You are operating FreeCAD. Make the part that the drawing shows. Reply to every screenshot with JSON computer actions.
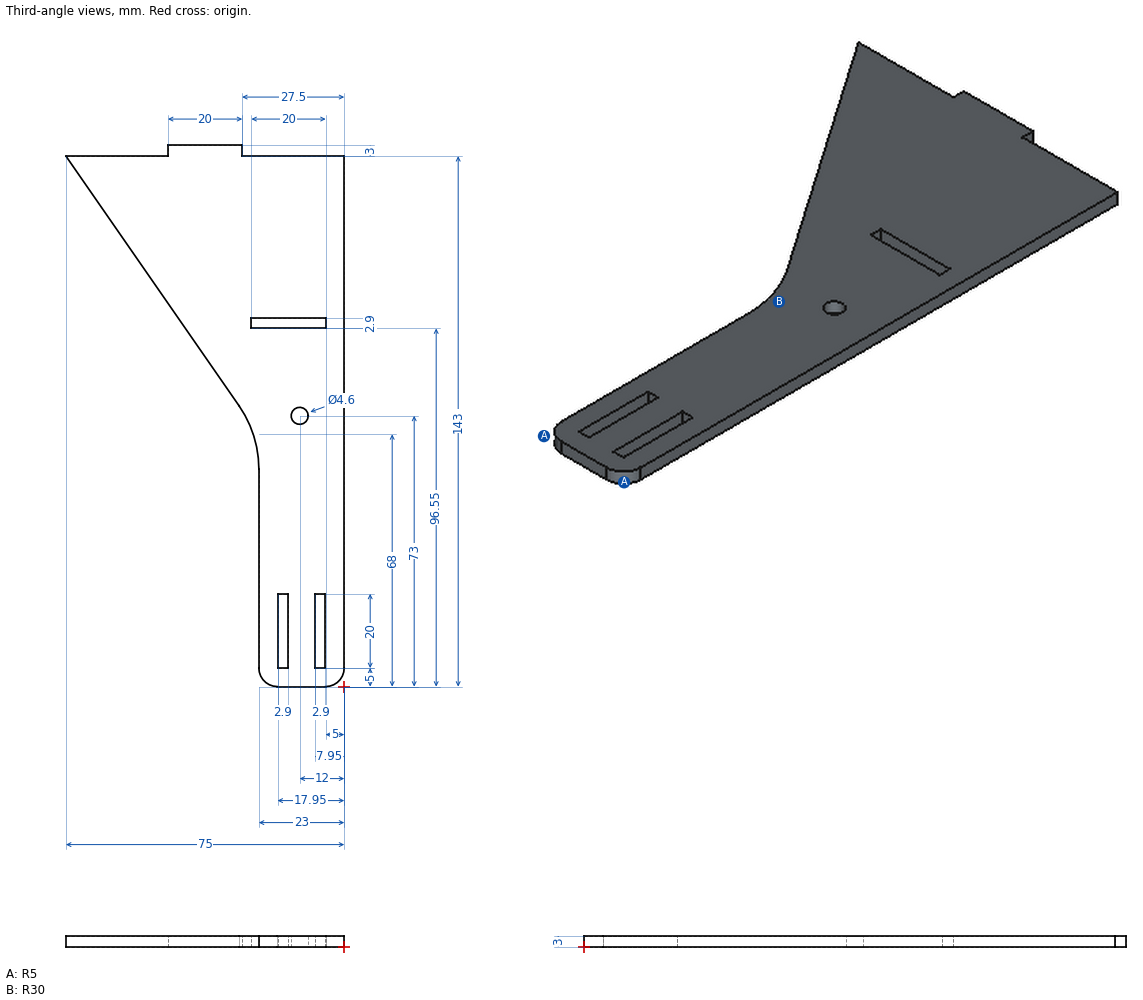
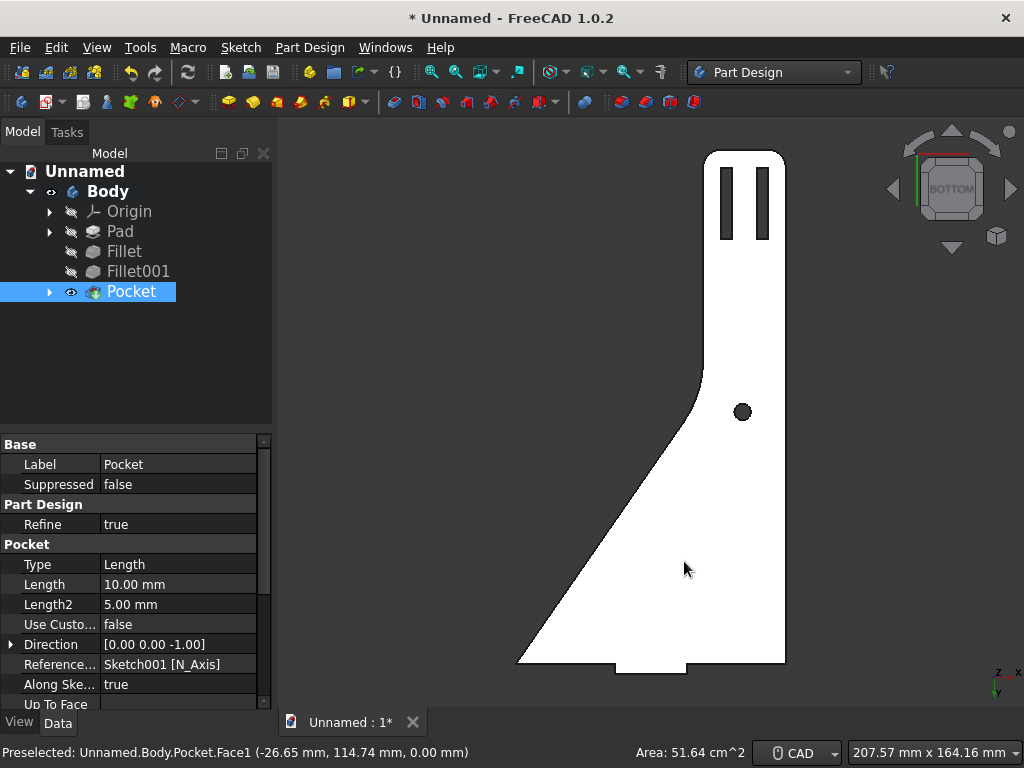
{"action": "left_click", "coordinate": [46, 102]}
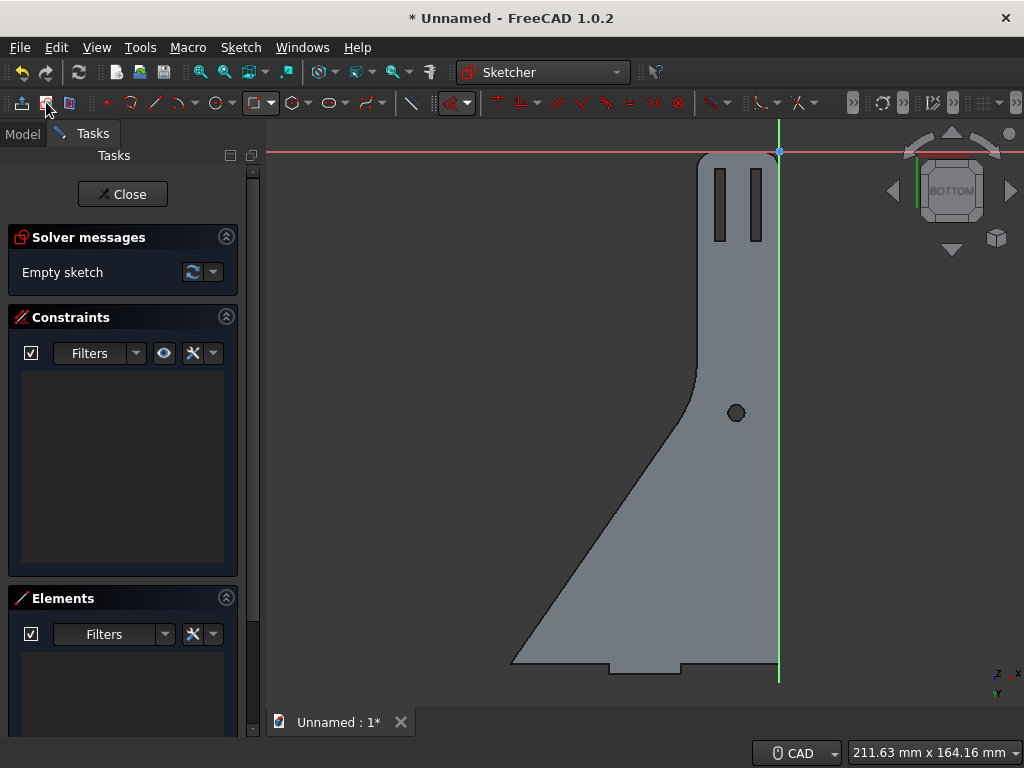
{"action": "scroll", "coordinate": [755, 520], "scroll_direction": "up", "scroll_amount": 9}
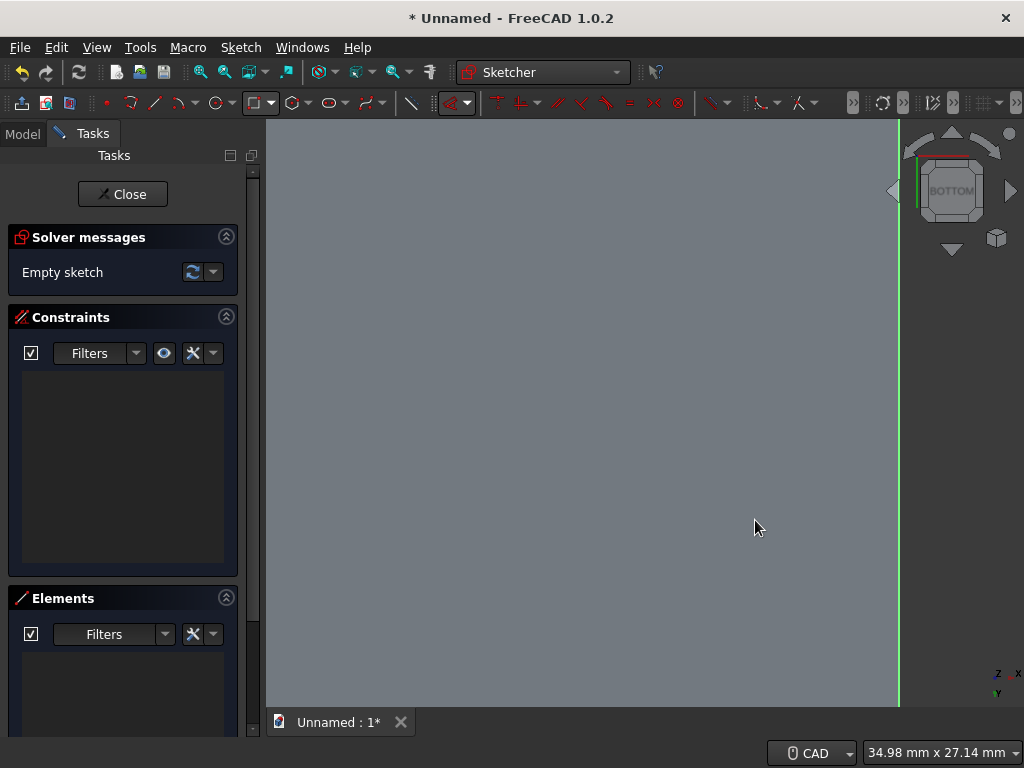
{"action": "left_click", "coordinate": [254, 104]}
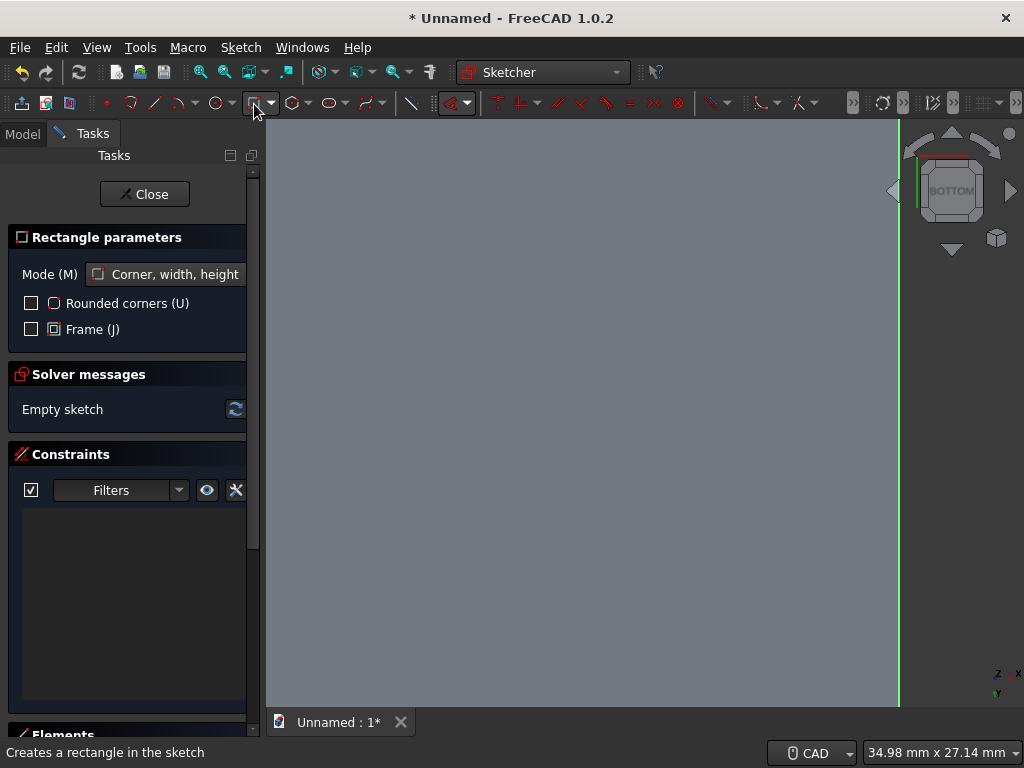
{"action": "left_click", "coordinate": [357, 380]}
{"action": "mouse_move", "coordinate": [791, 442]}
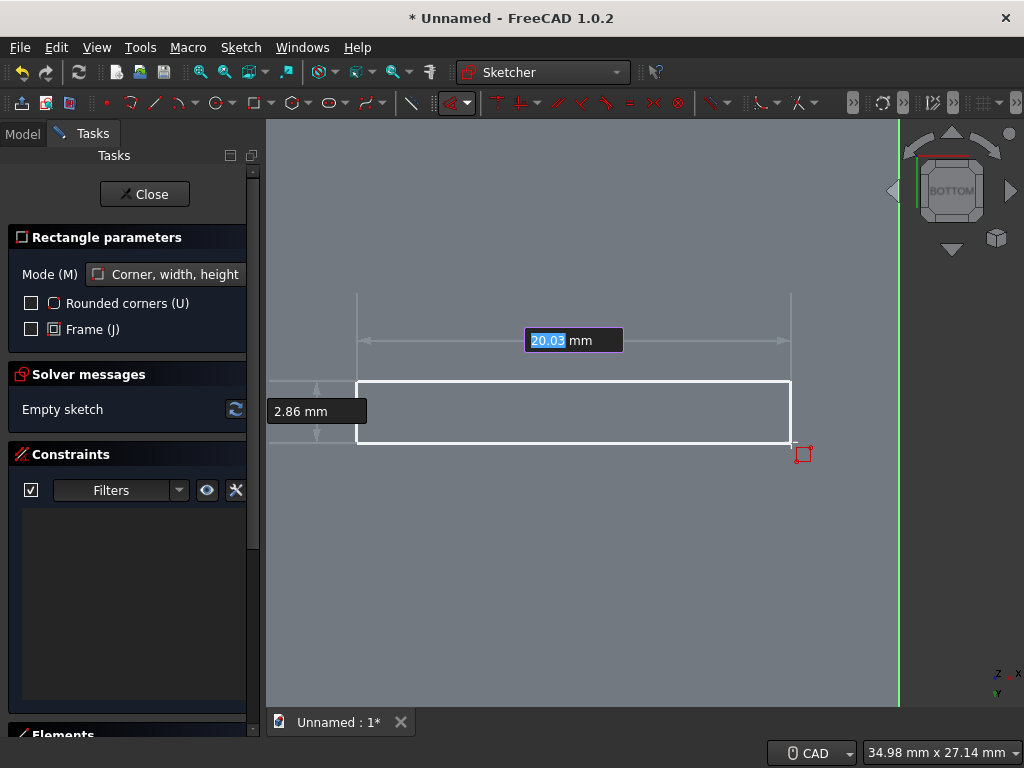
{"action": "type", "text": "20"}
{"action": "key", "text": "Tab"}
{"action": "type", "text": "2.9"}
{"action": "key", "text": "Return"}
{"action": "key", "text": "Escape"}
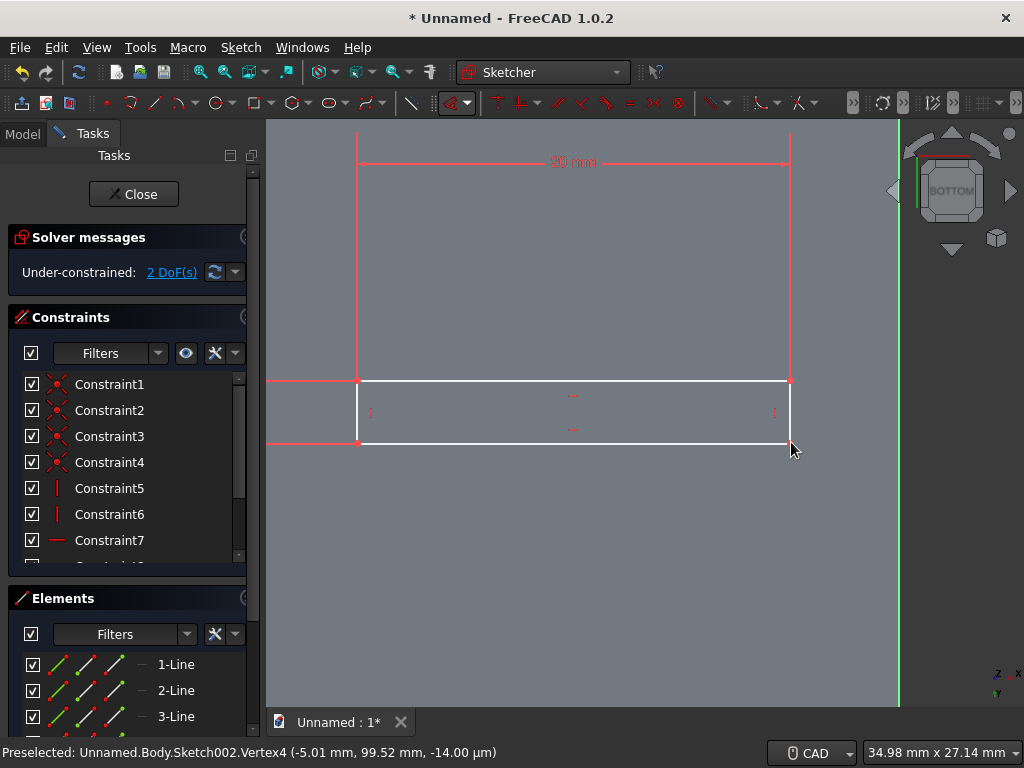
{"action": "left_click", "coordinate": [790, 444]}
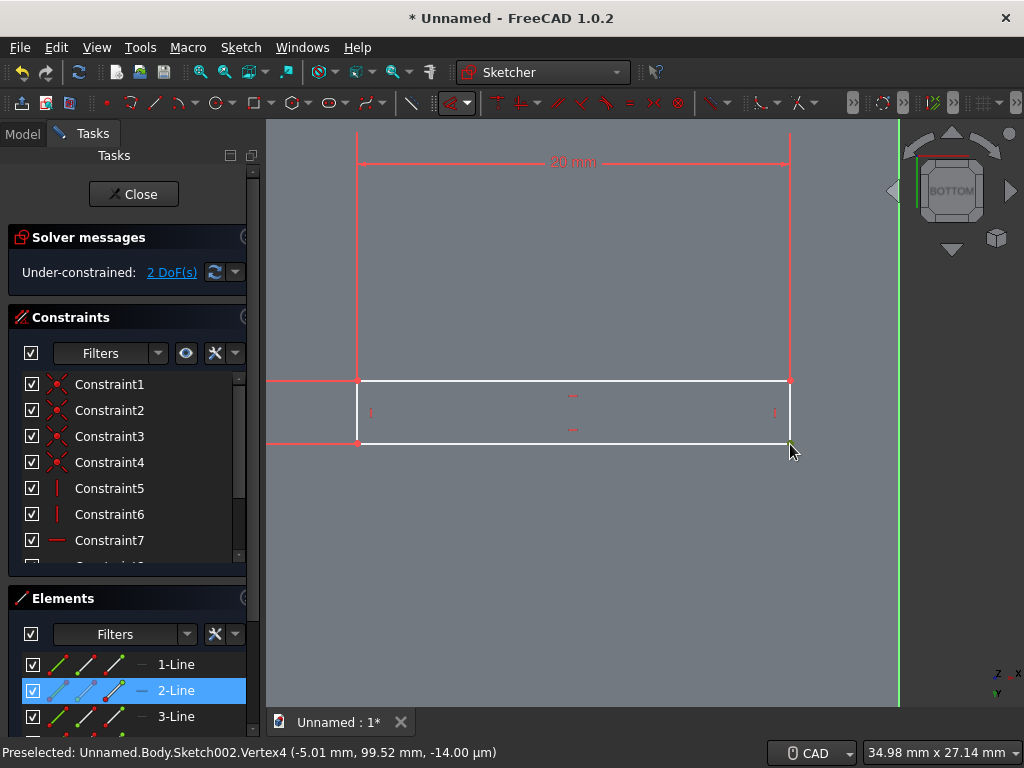
{"action": "key", "text": "l"}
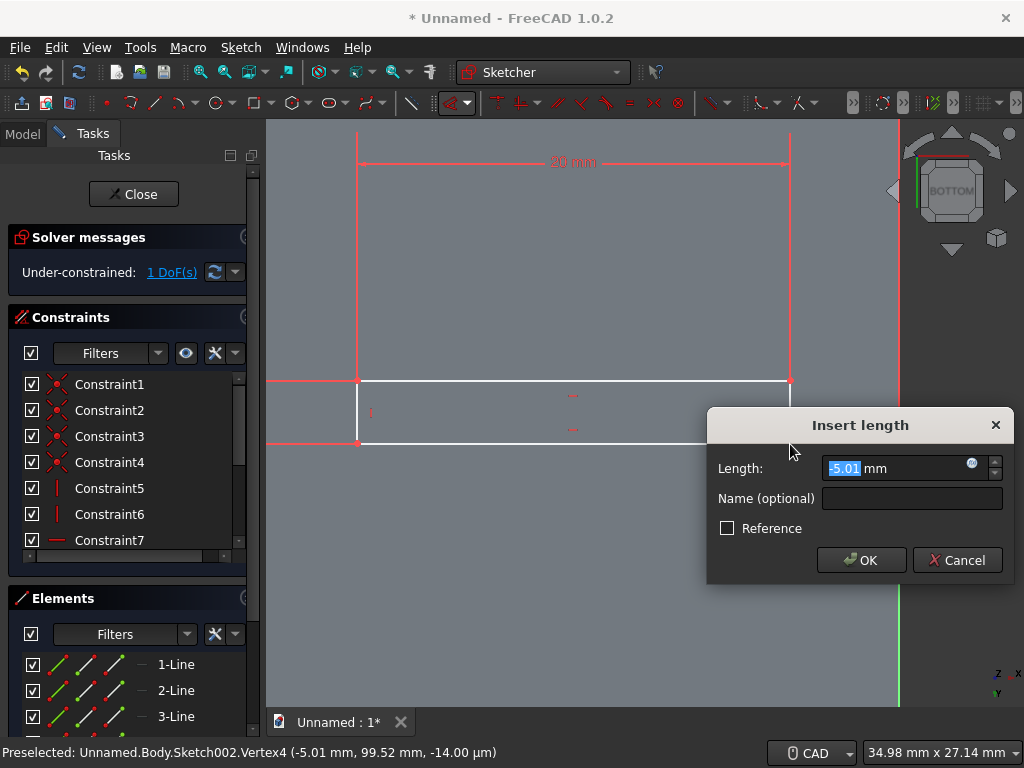
{"action": "type", "text": "-5"}
{"action": "key", "text": "Return"}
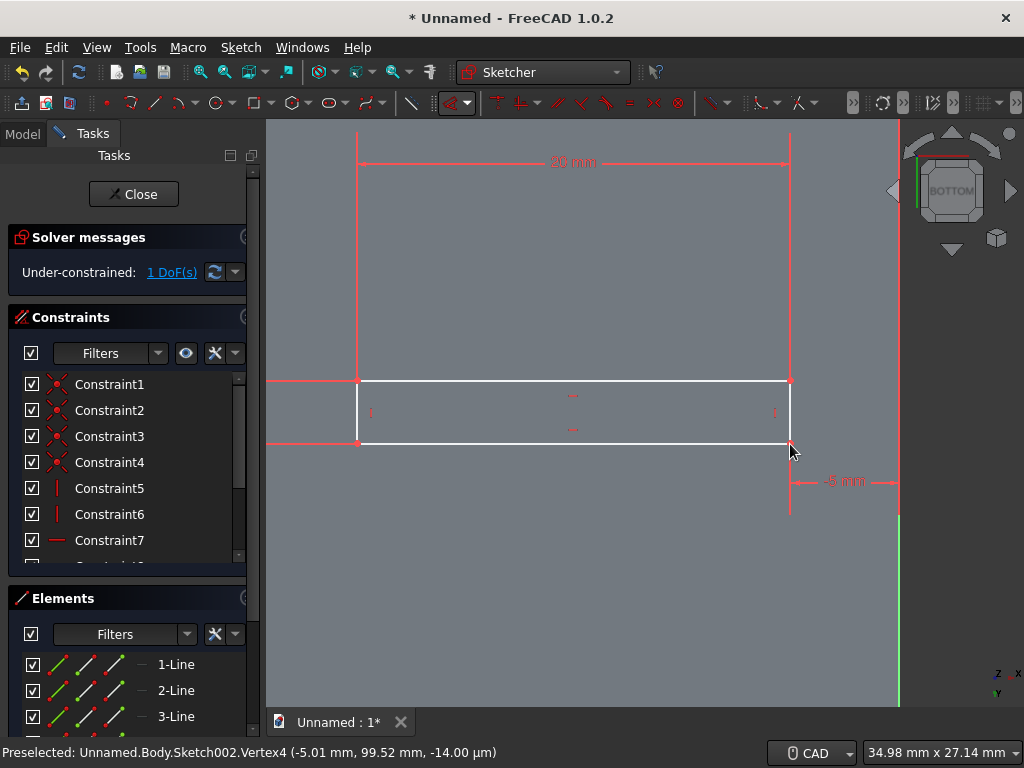
{"action": "left_click", "coordinate": [357, 381]}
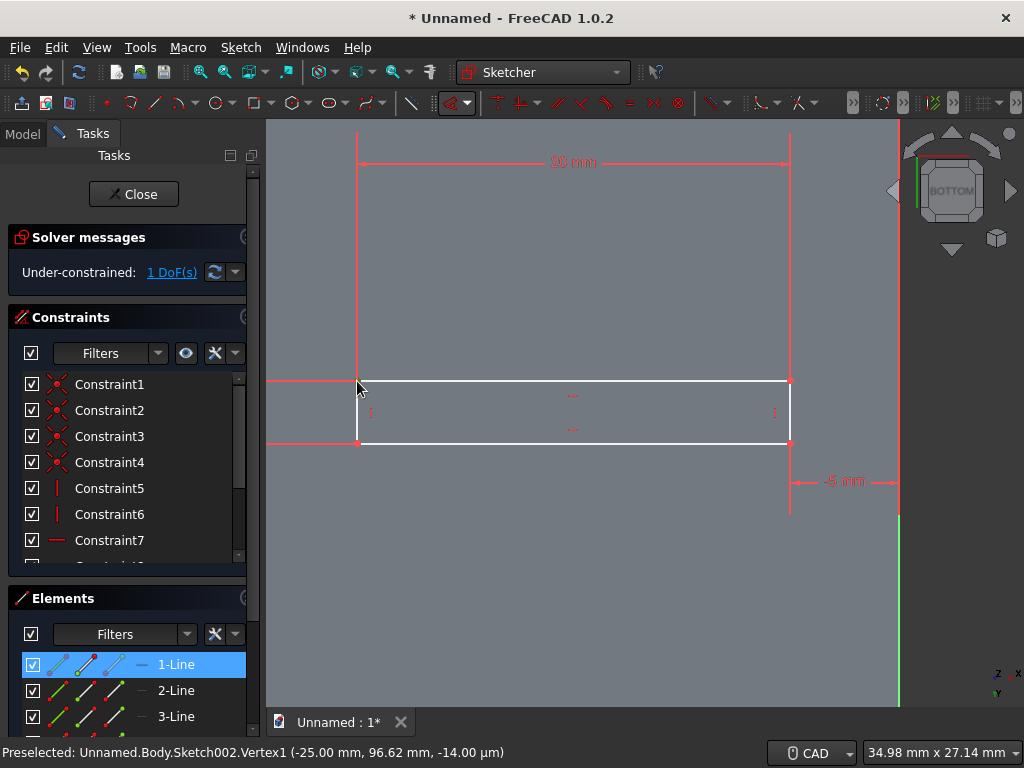
{"action": "left_click", "coordinate": [470, 104]}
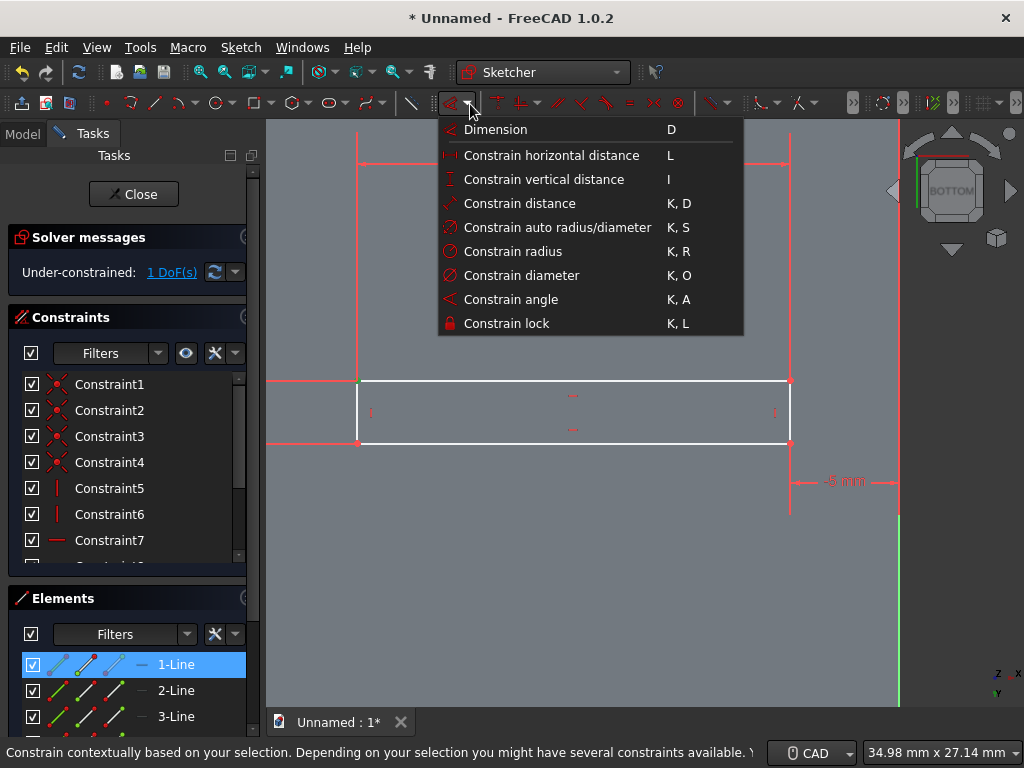
{"action": "left_click", "coordinate": [591, 179]}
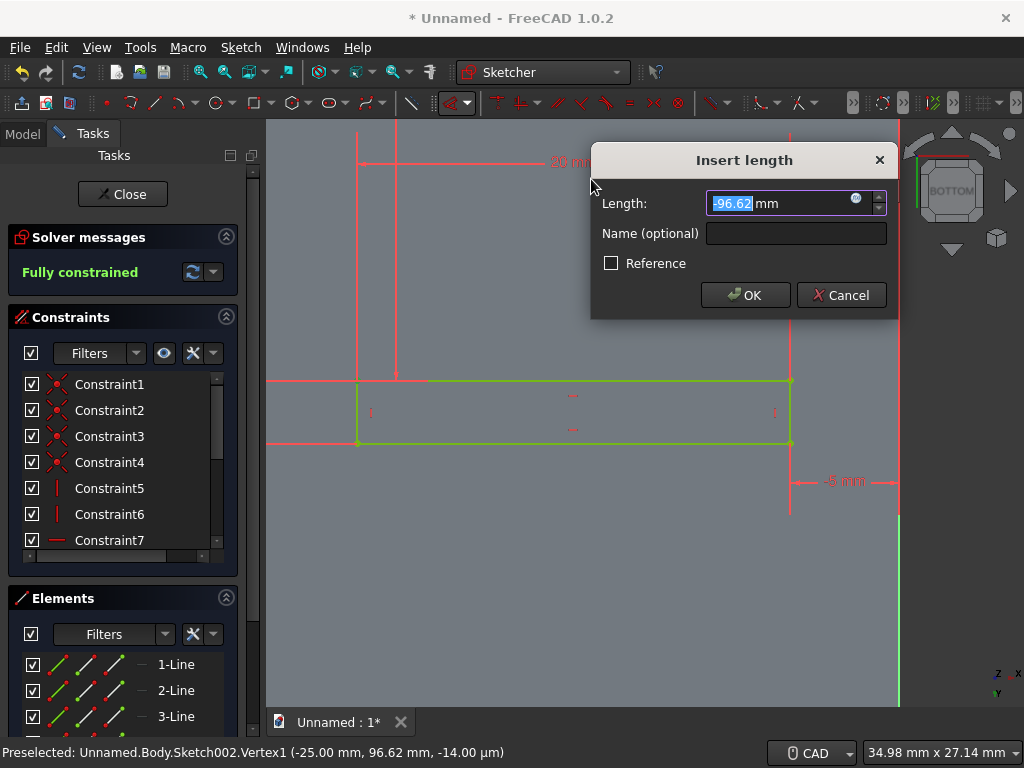
{"action": "type", "text": "-96.55"}
{"action": "key", "text": "Return"}